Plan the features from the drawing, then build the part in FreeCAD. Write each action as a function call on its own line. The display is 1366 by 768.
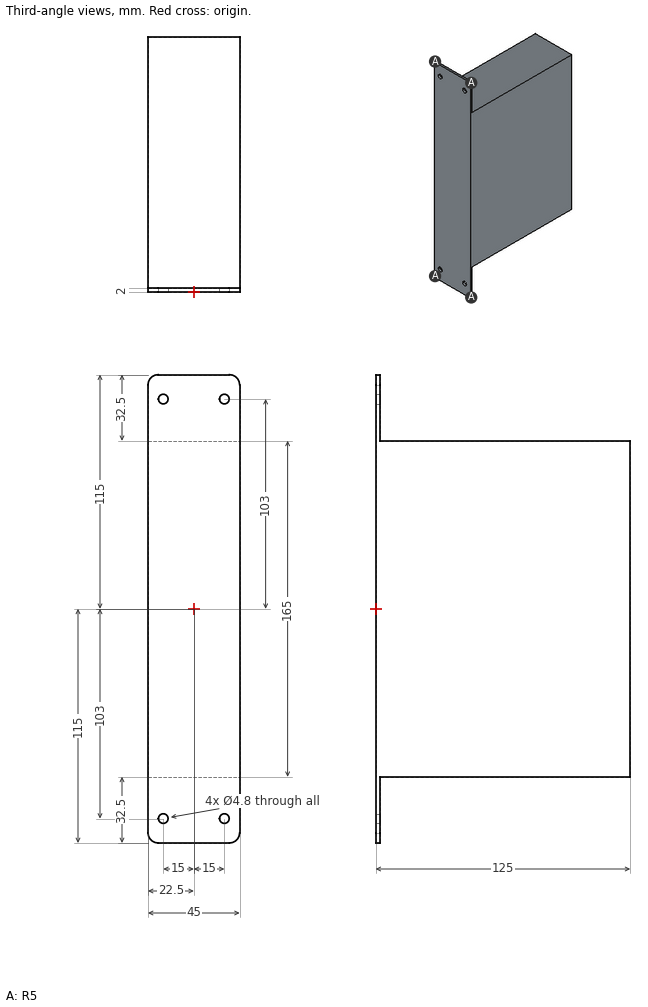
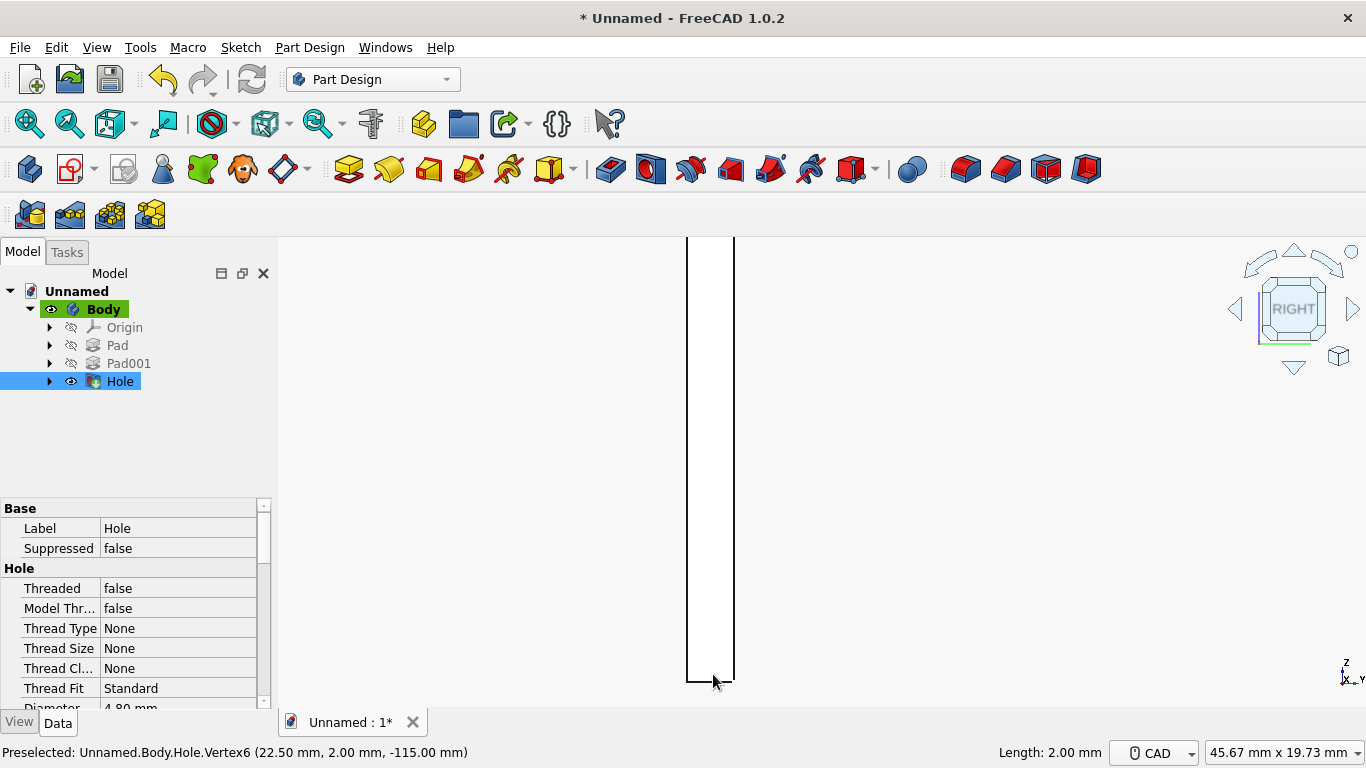
click(30, 124)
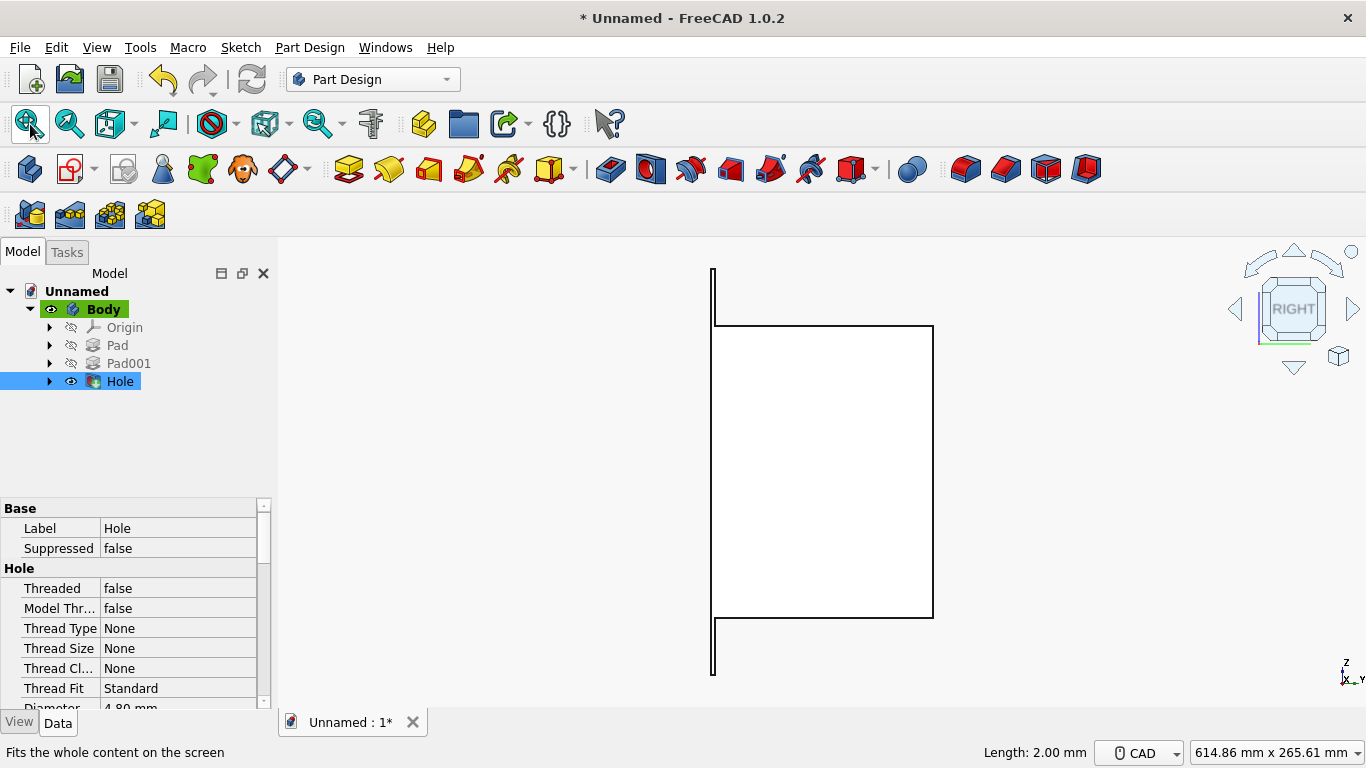
key(5)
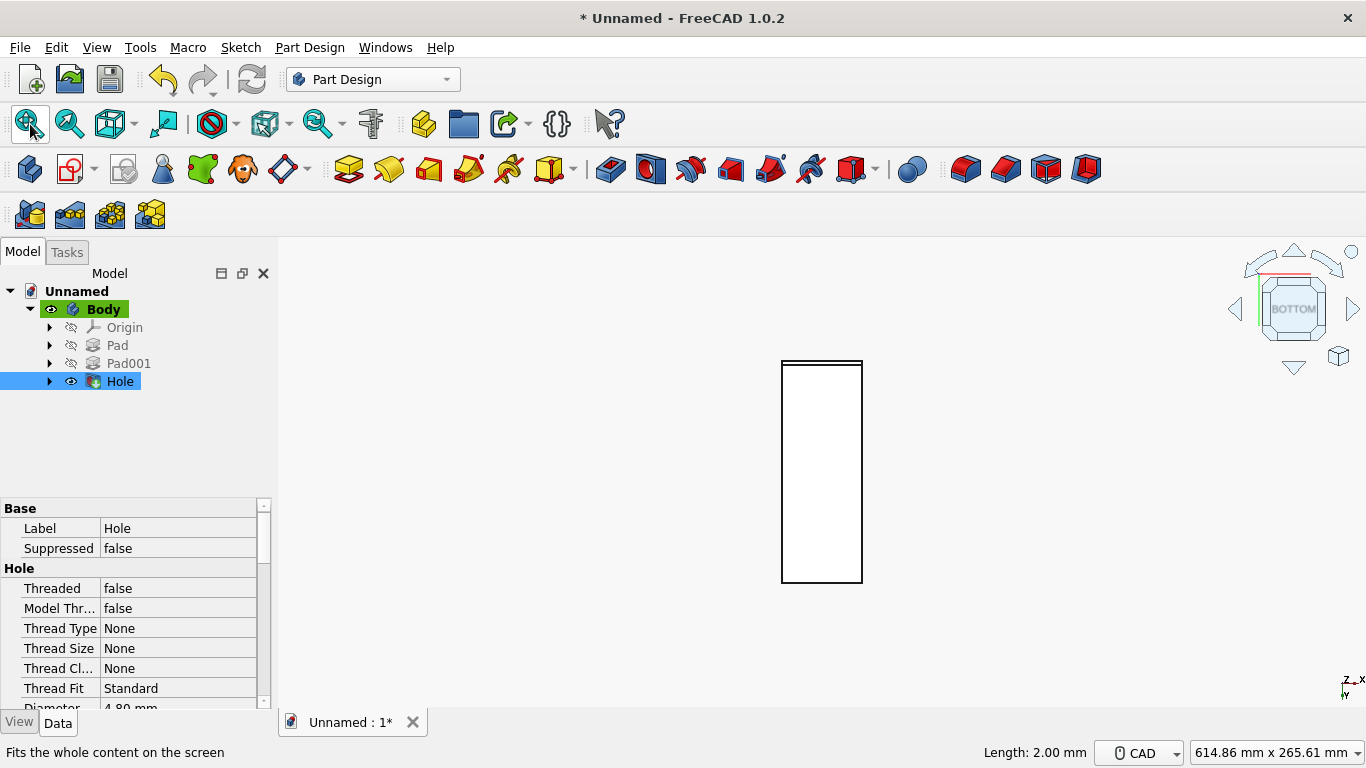
scroll(782, 362, up, 13)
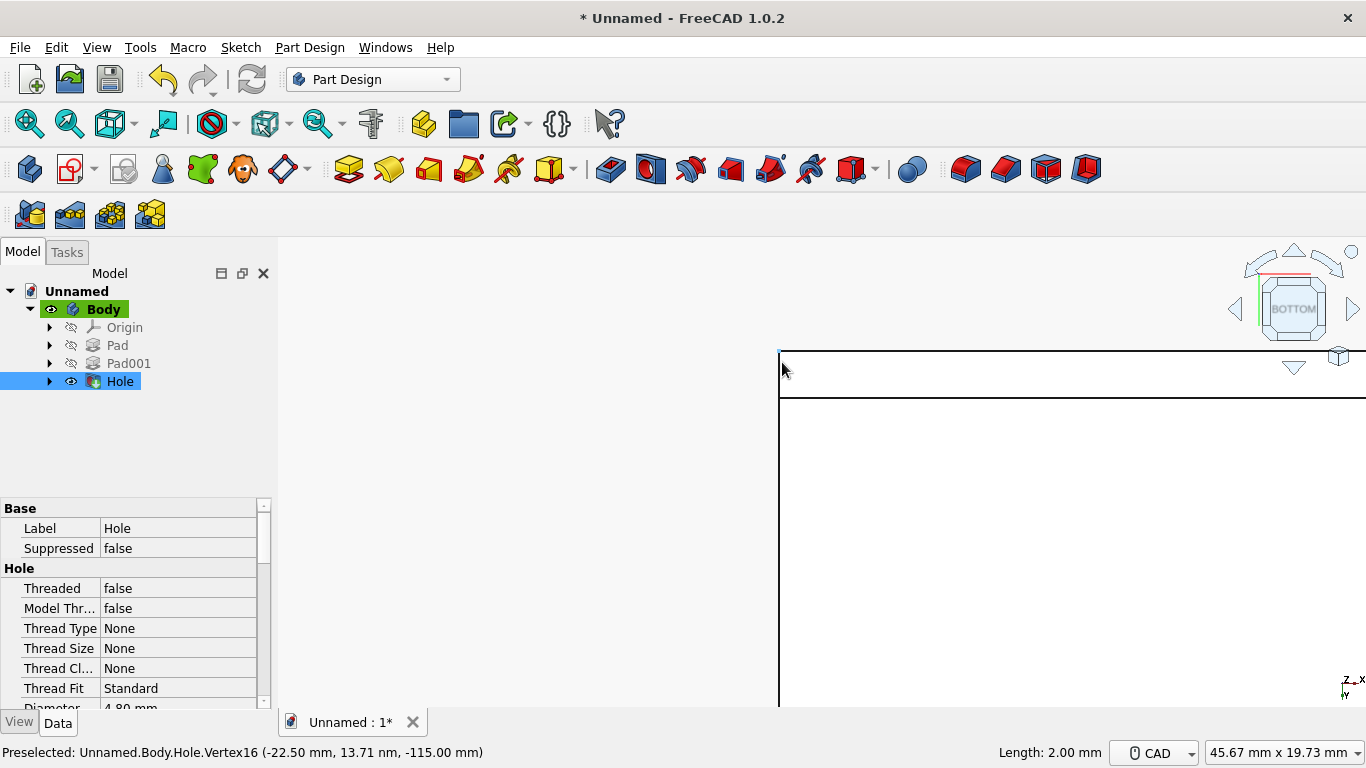
click(779, 374, ctrl)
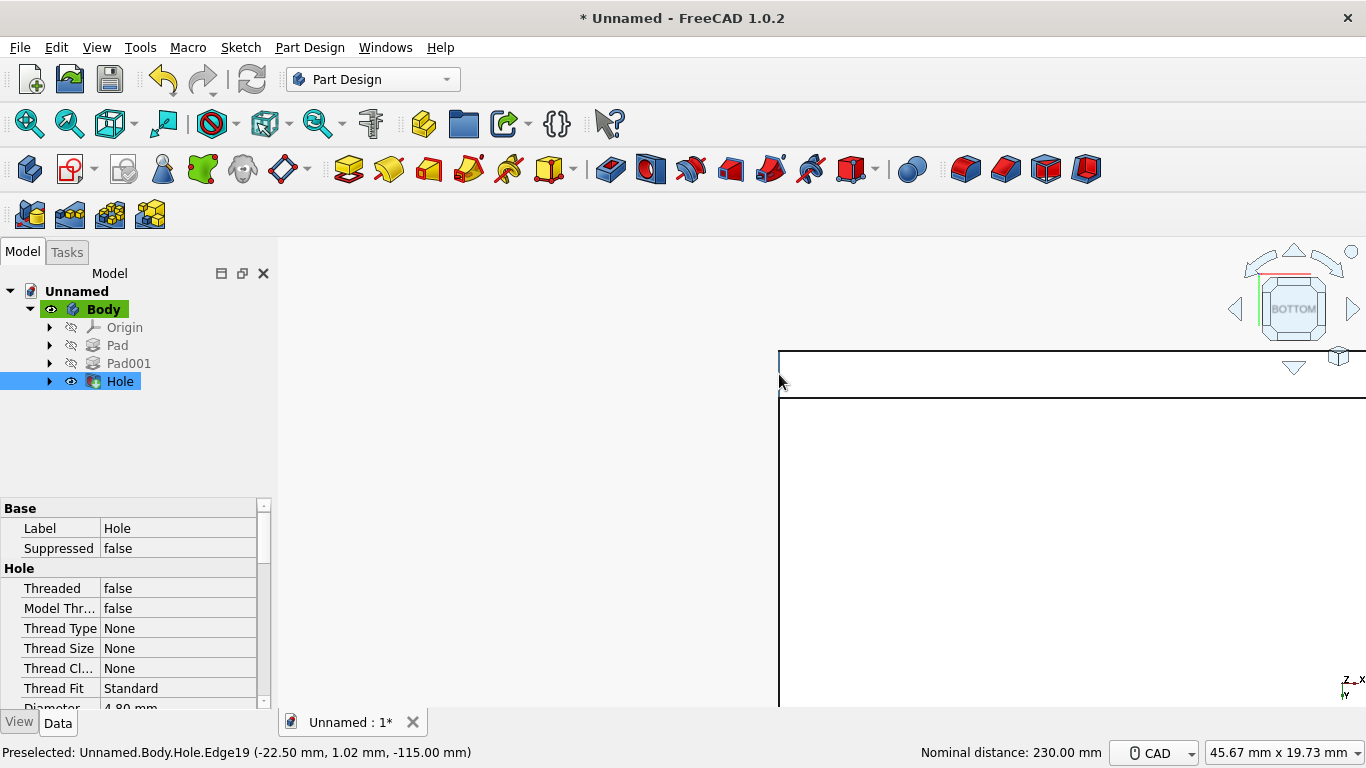
click(30, 124)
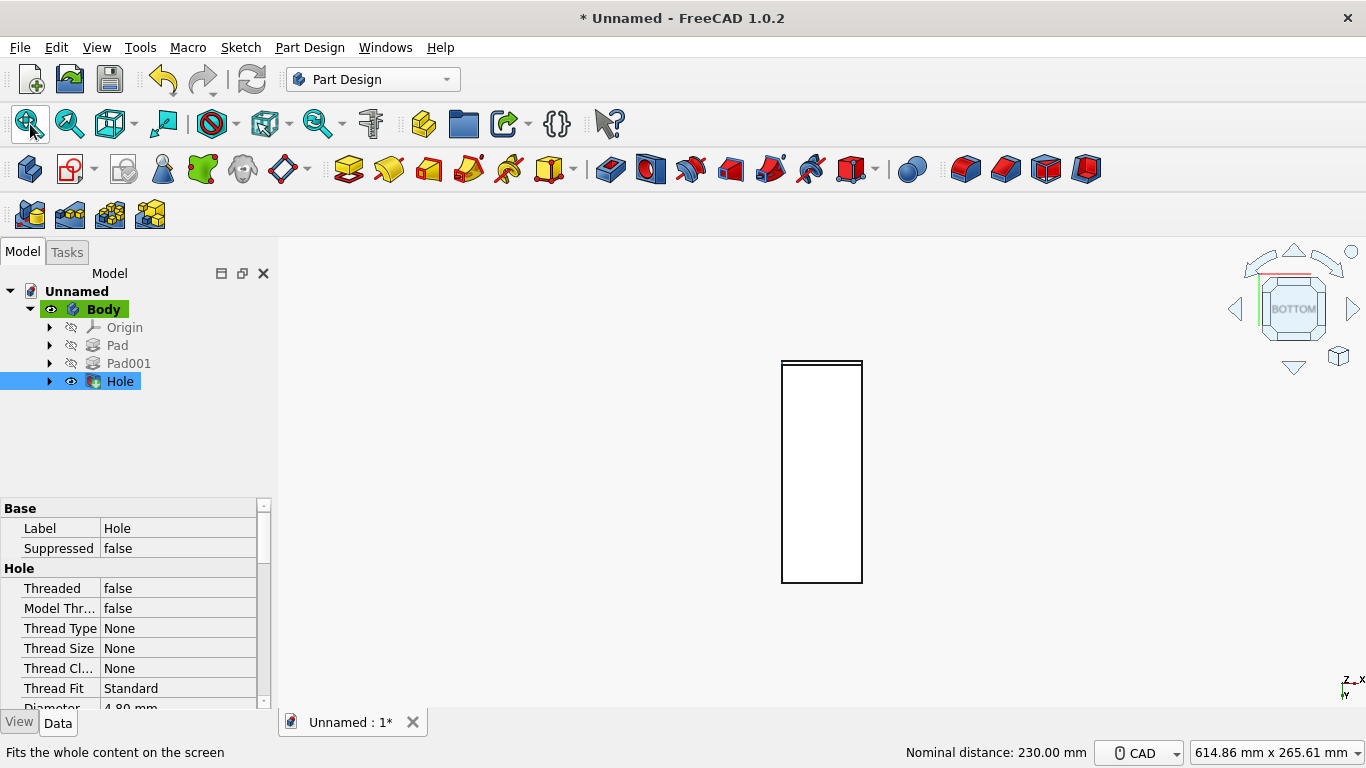
key(4)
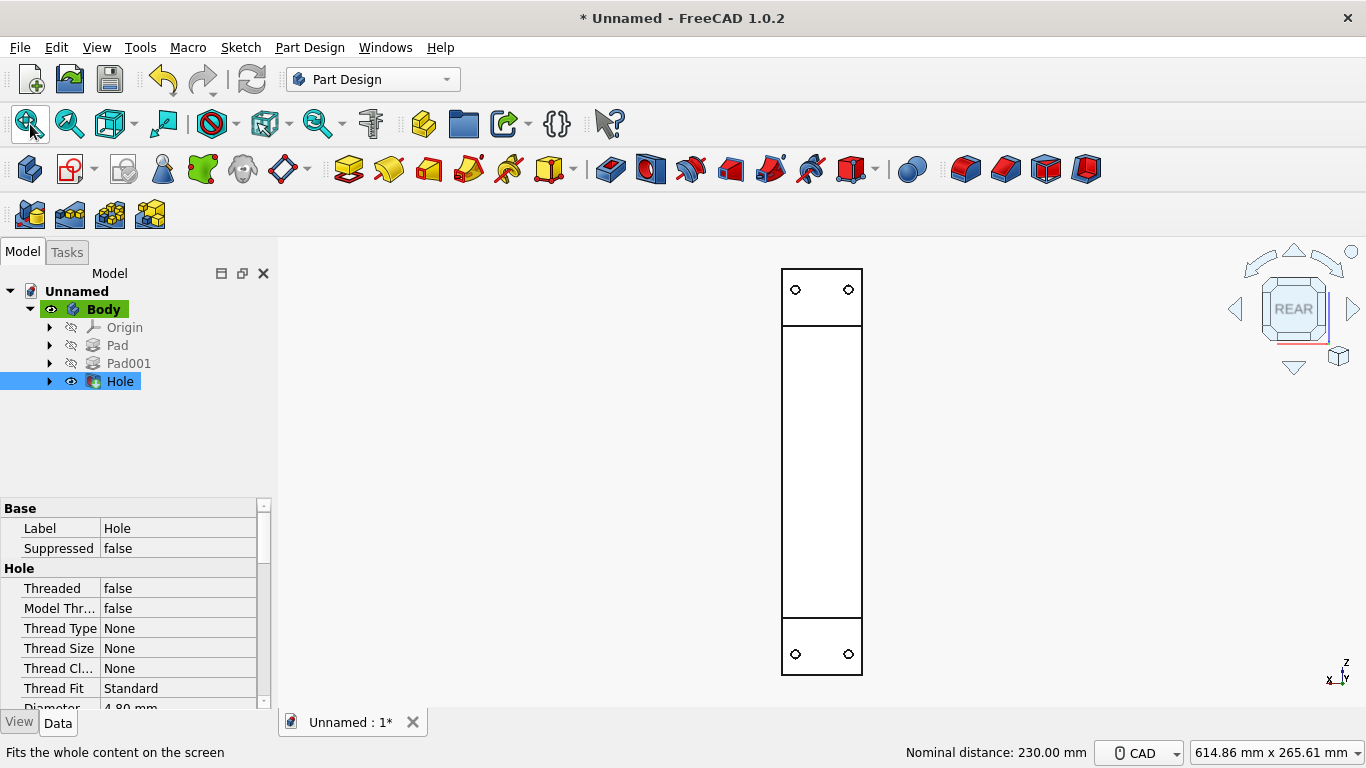
scroll(782, 674, up, 13)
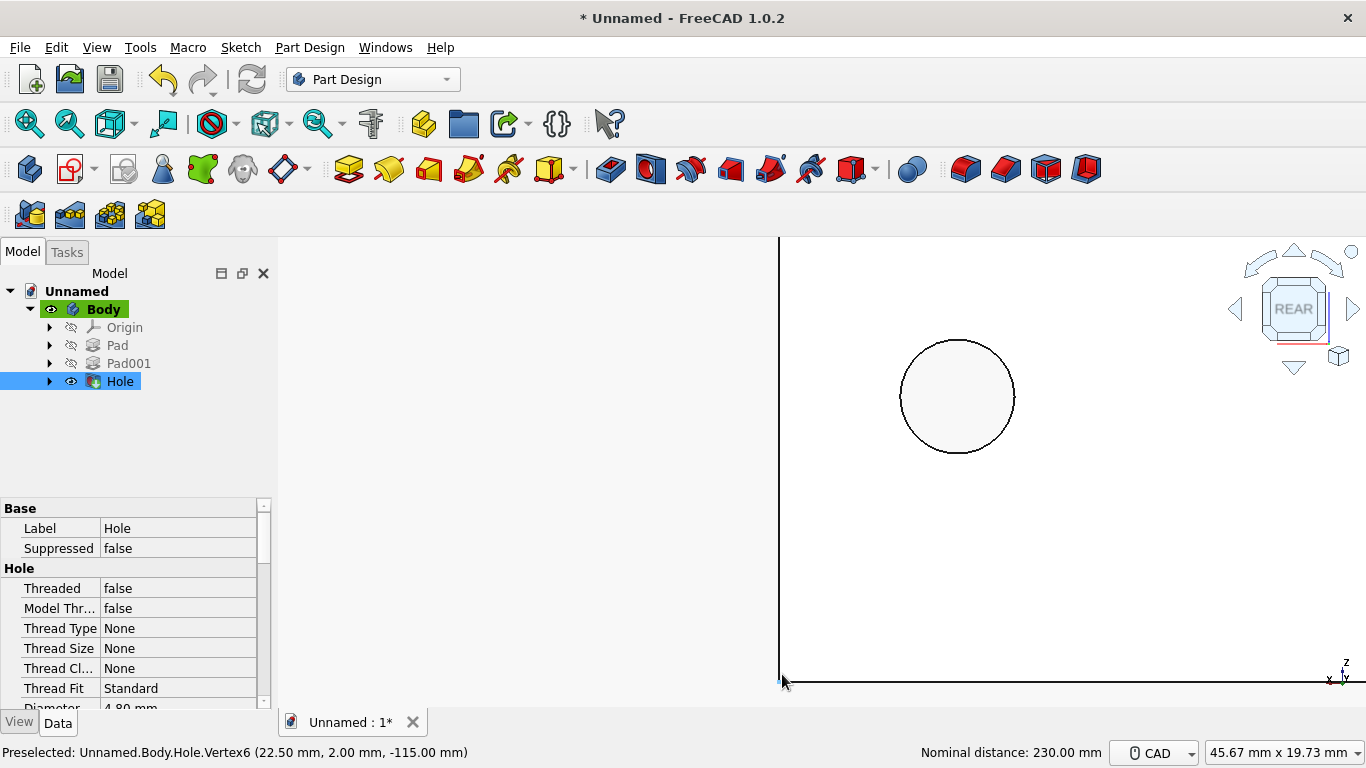
click(30, 124)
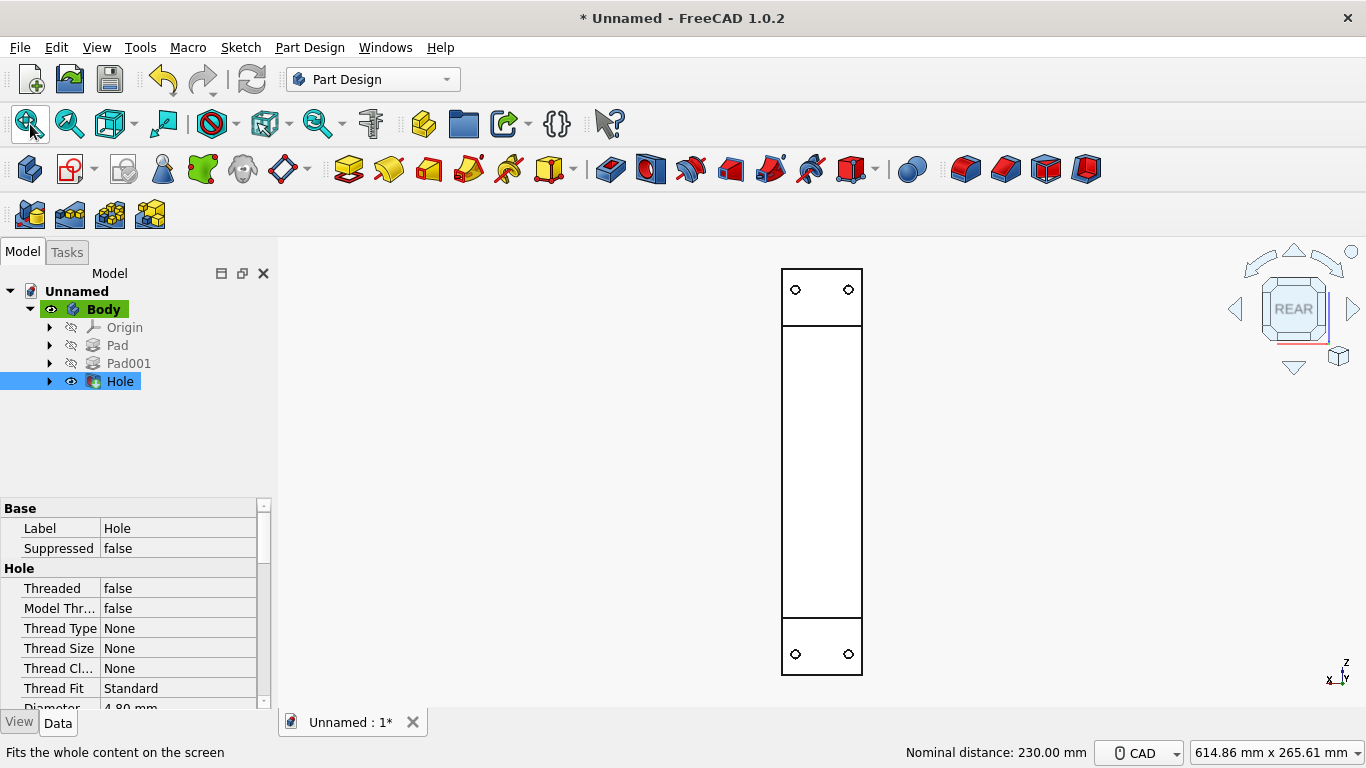
key(6)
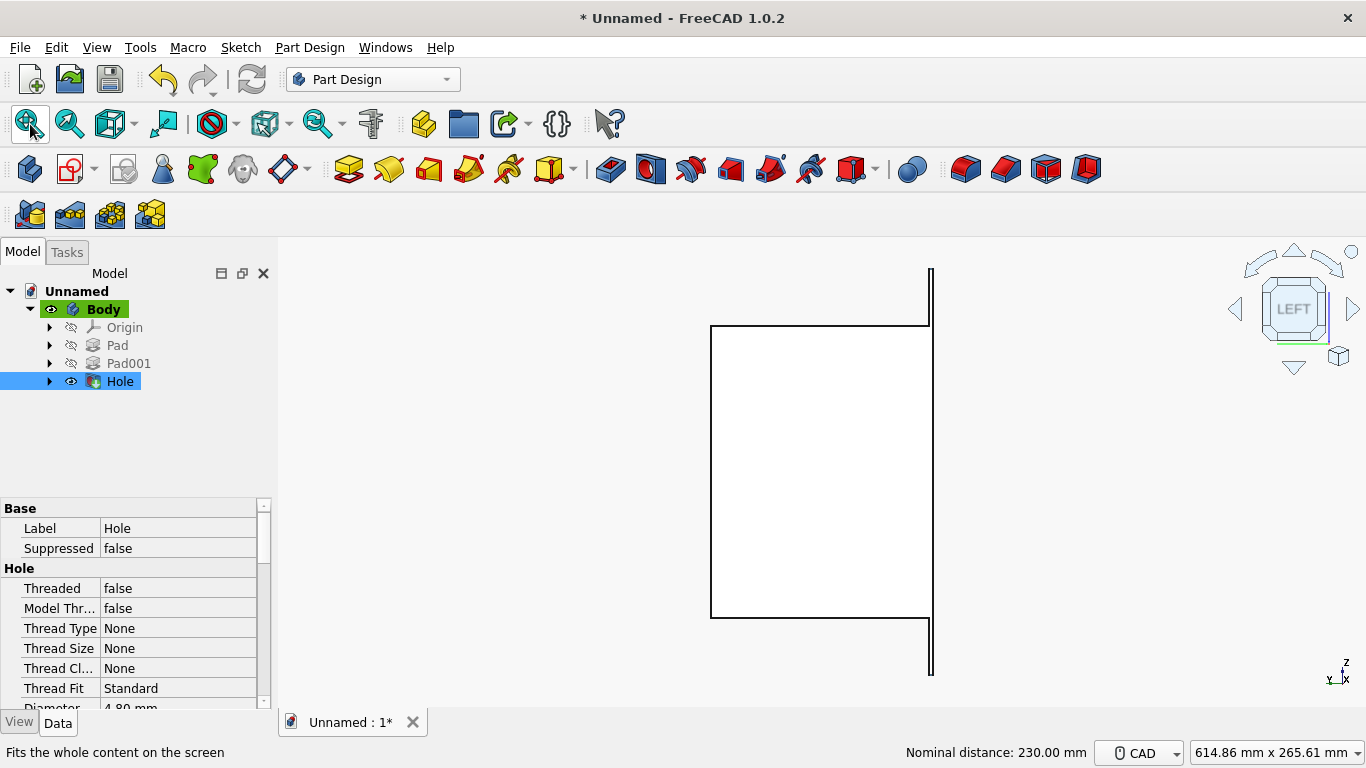
scroll(931, 674, up, 13)